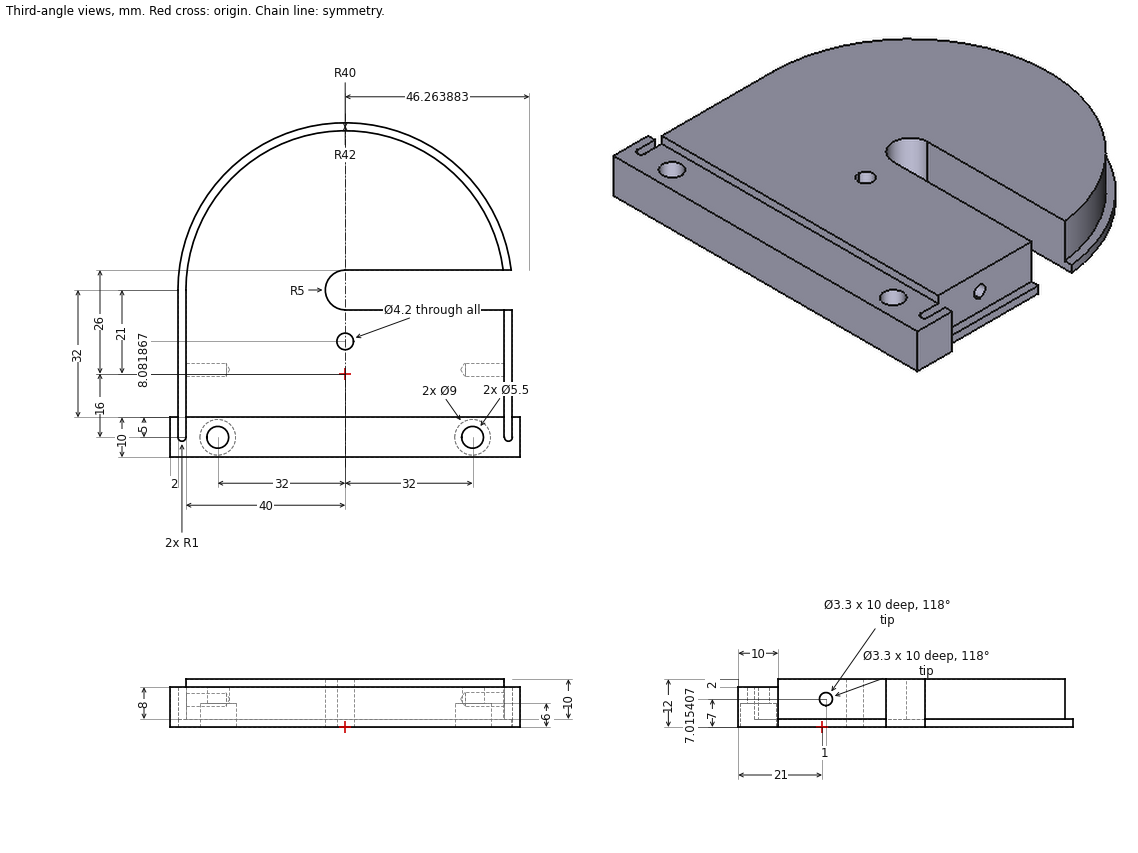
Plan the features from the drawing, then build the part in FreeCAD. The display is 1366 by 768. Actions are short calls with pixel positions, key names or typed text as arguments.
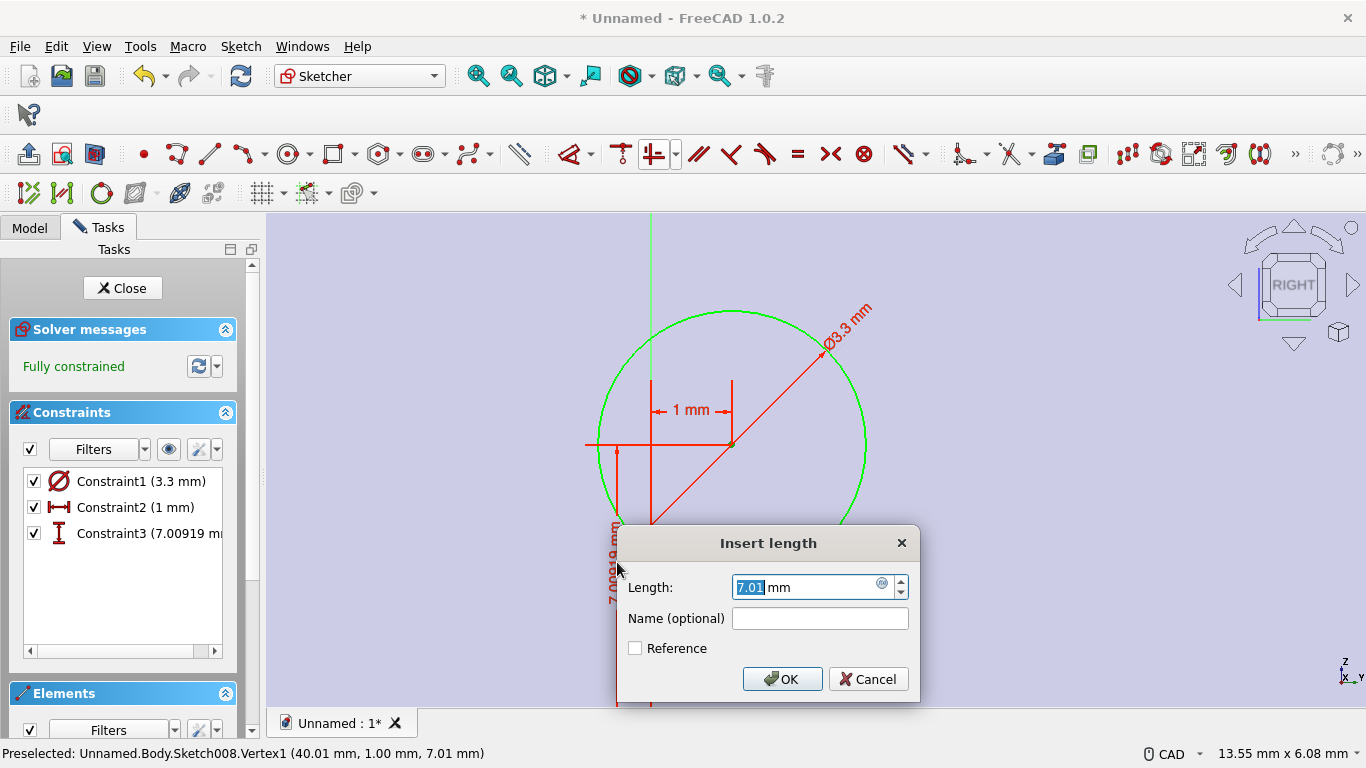
text(7.015407)
key(Return)
key(Escape)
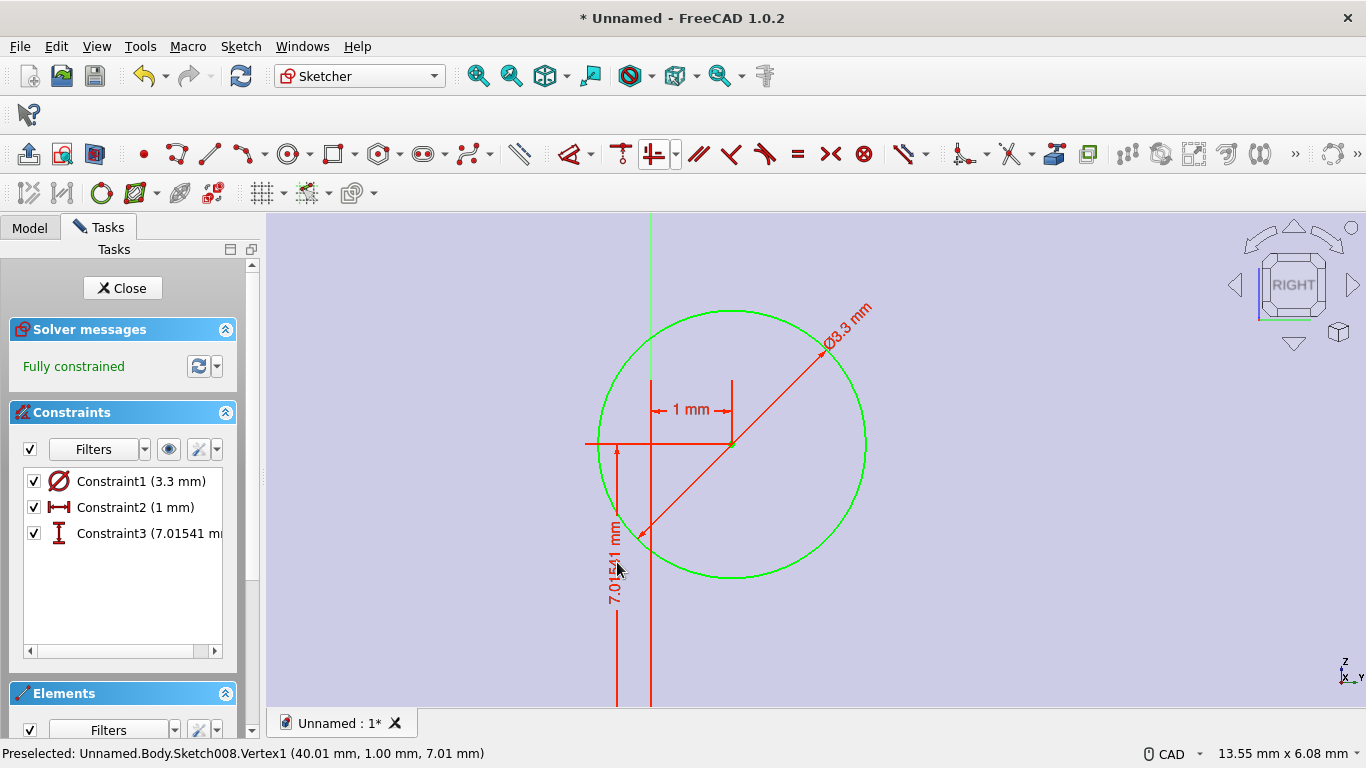
click(123, 288)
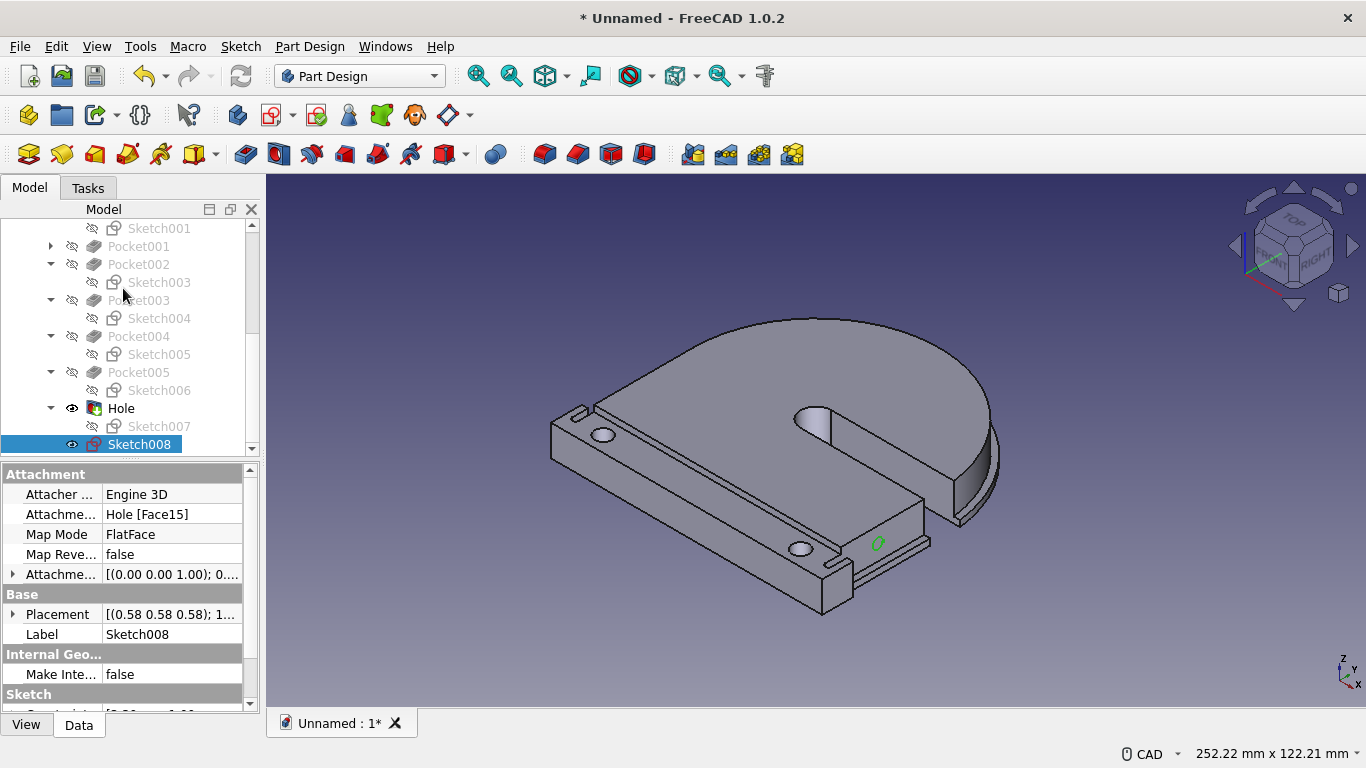
click(279, 154)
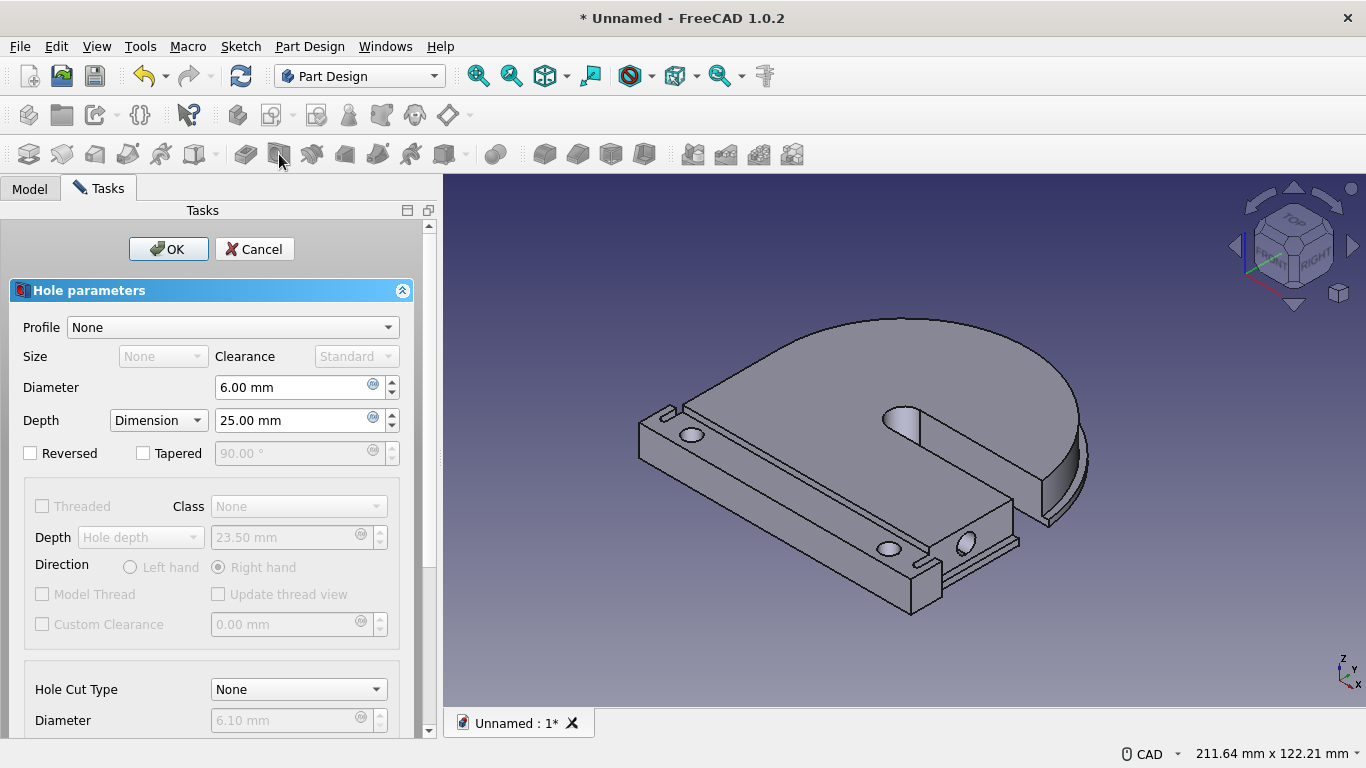
triple_click(300, 388)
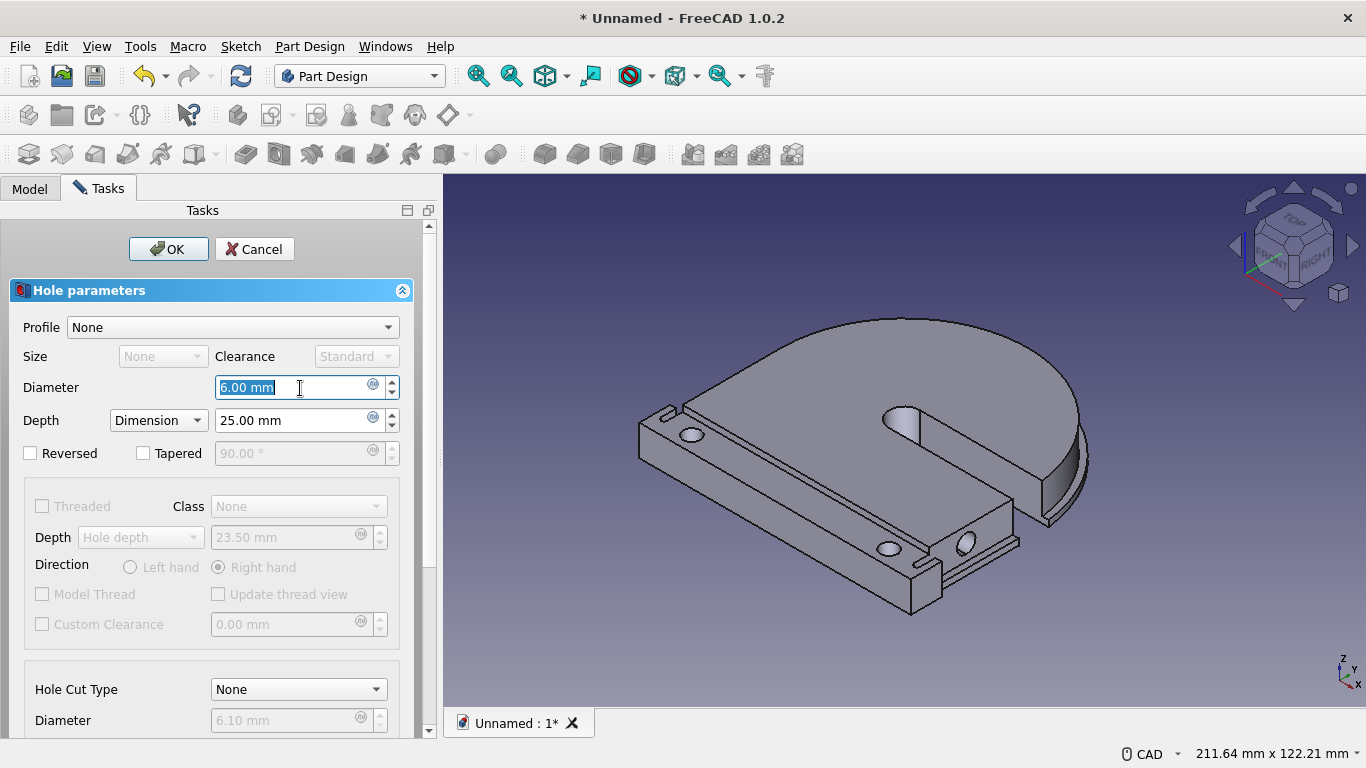
text(3.3)
key(Tab)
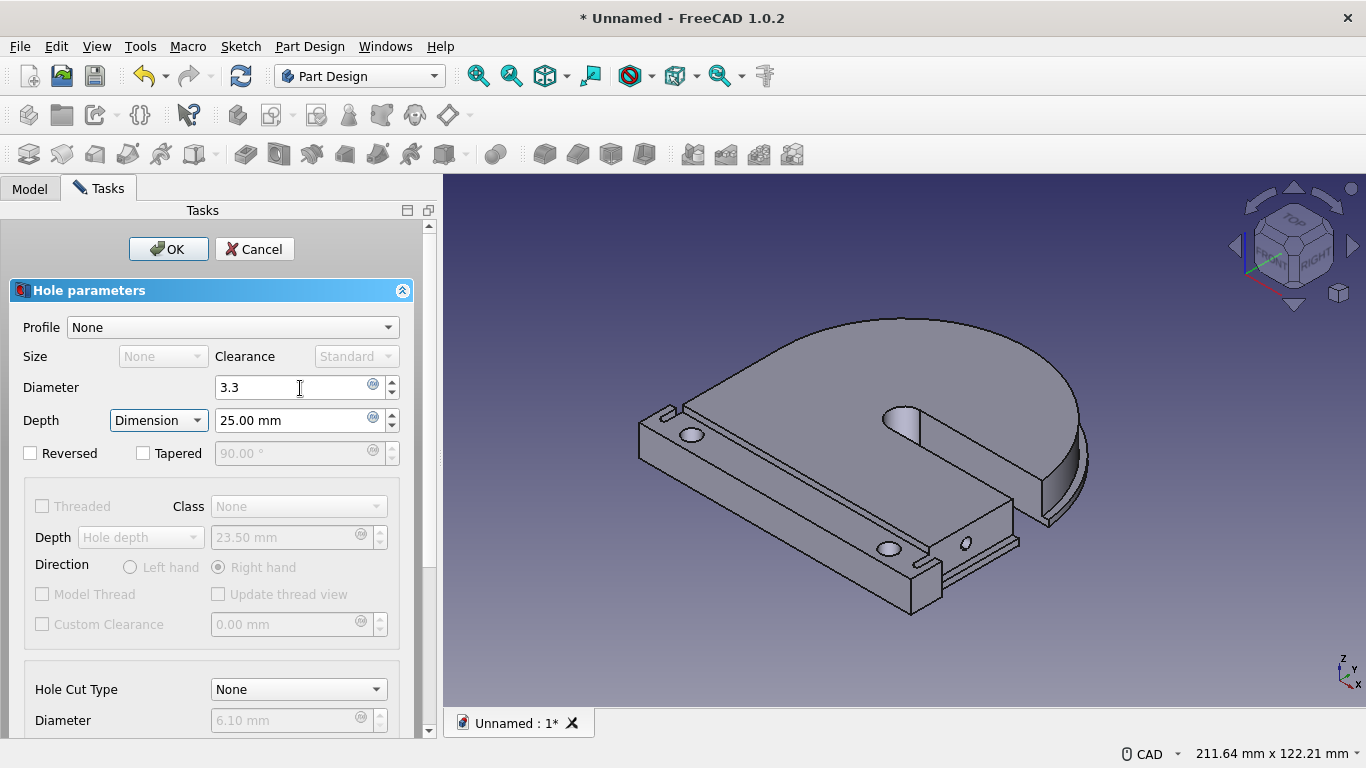
triple_click(300, 420)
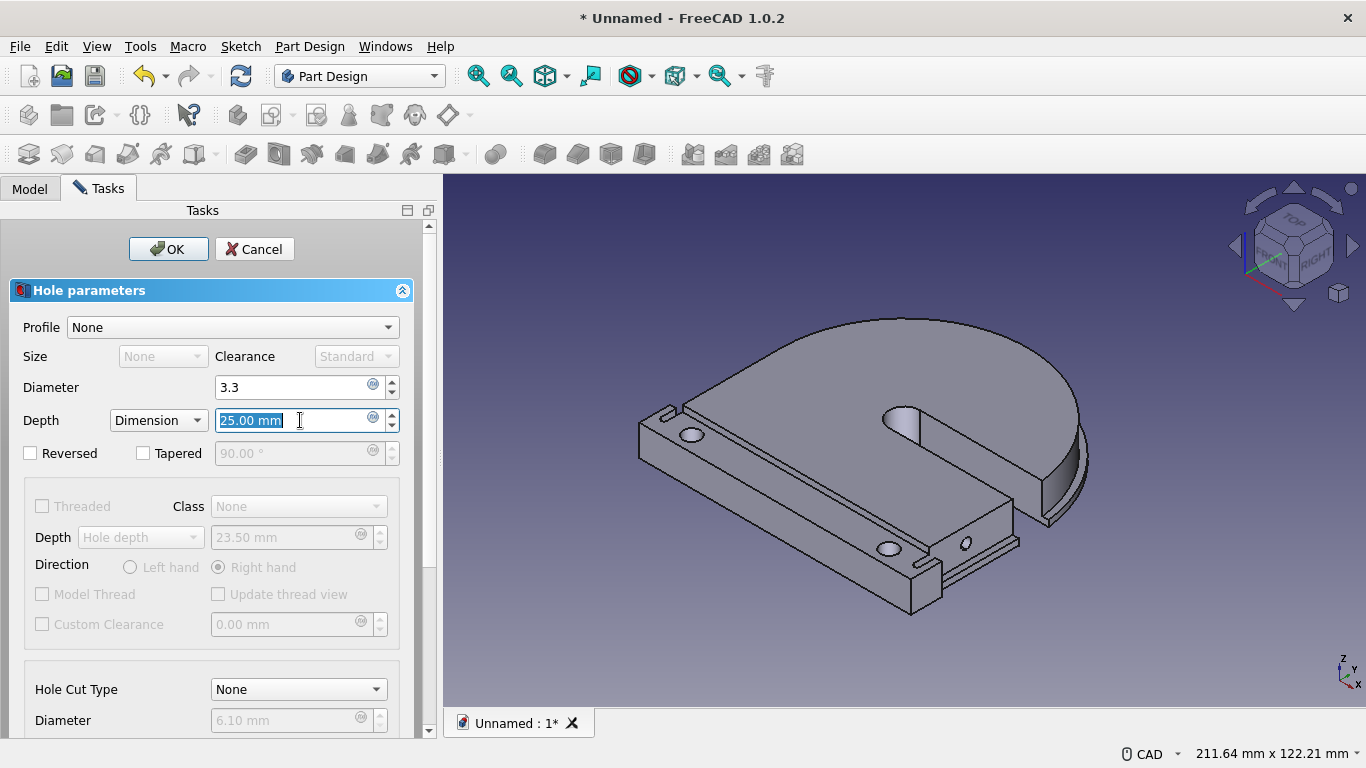
text(10)
key(Tab)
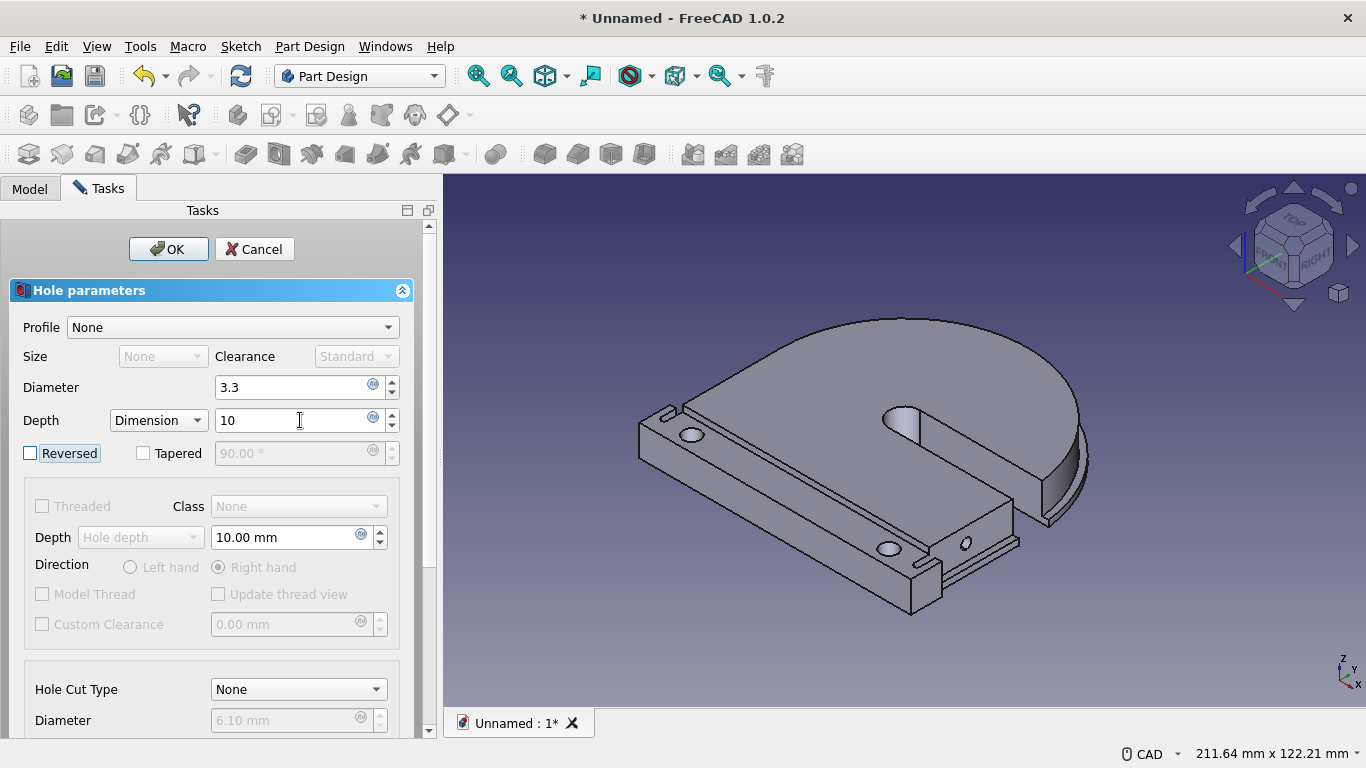
click(169, 249)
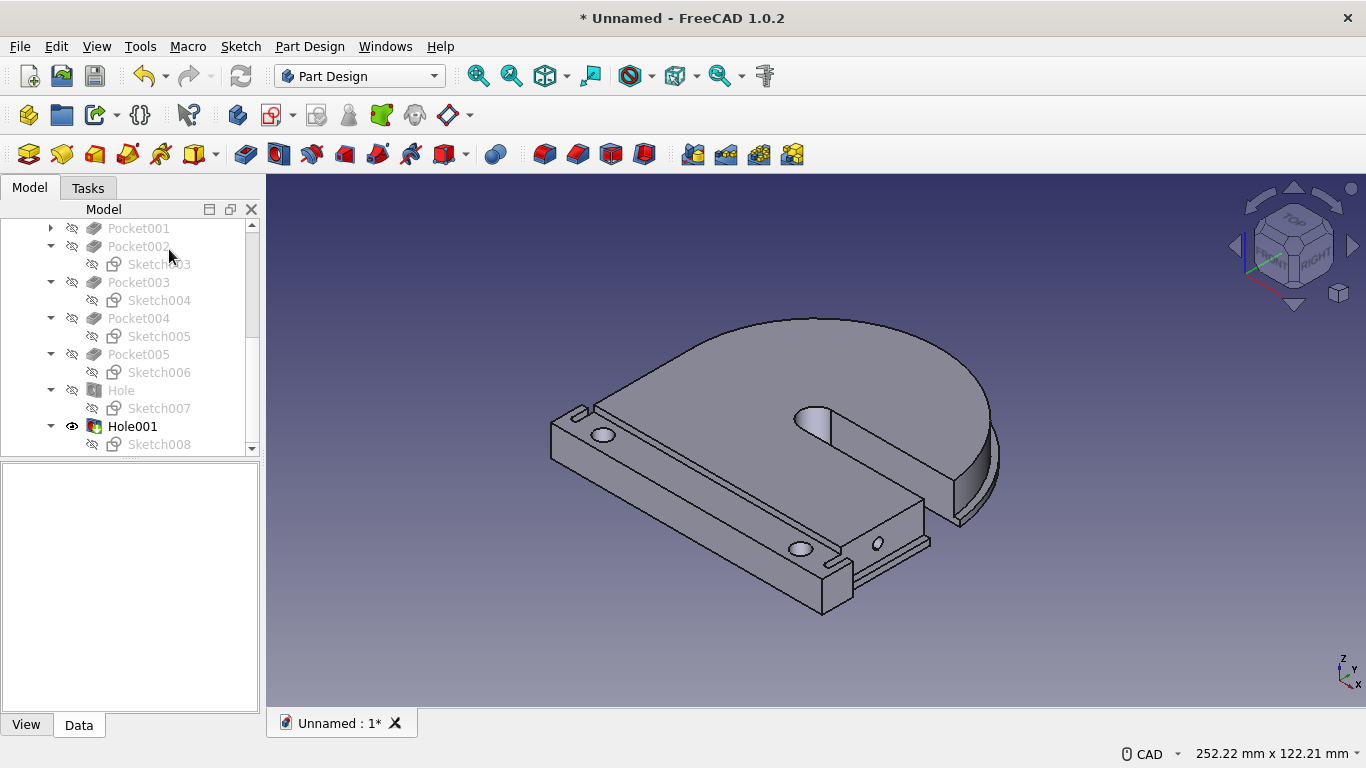
key(5)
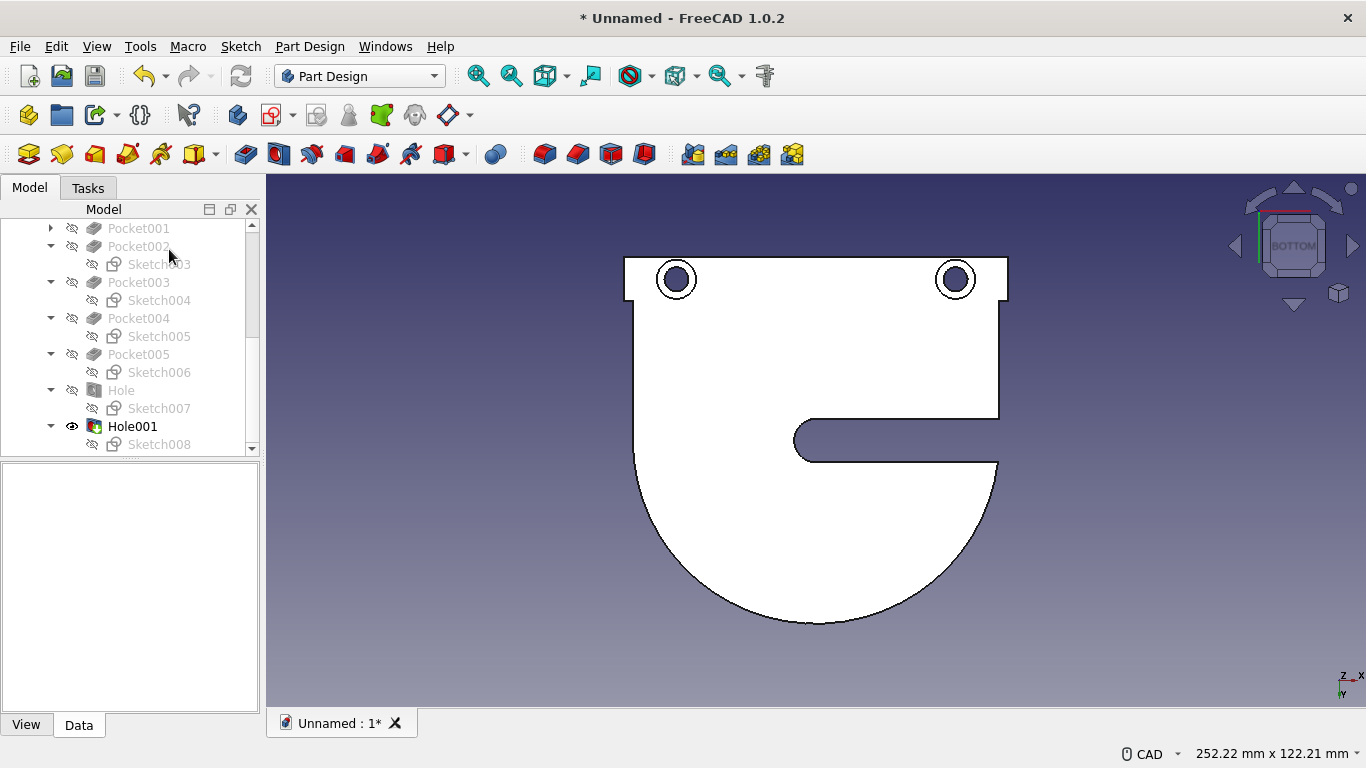
click(816, 544)